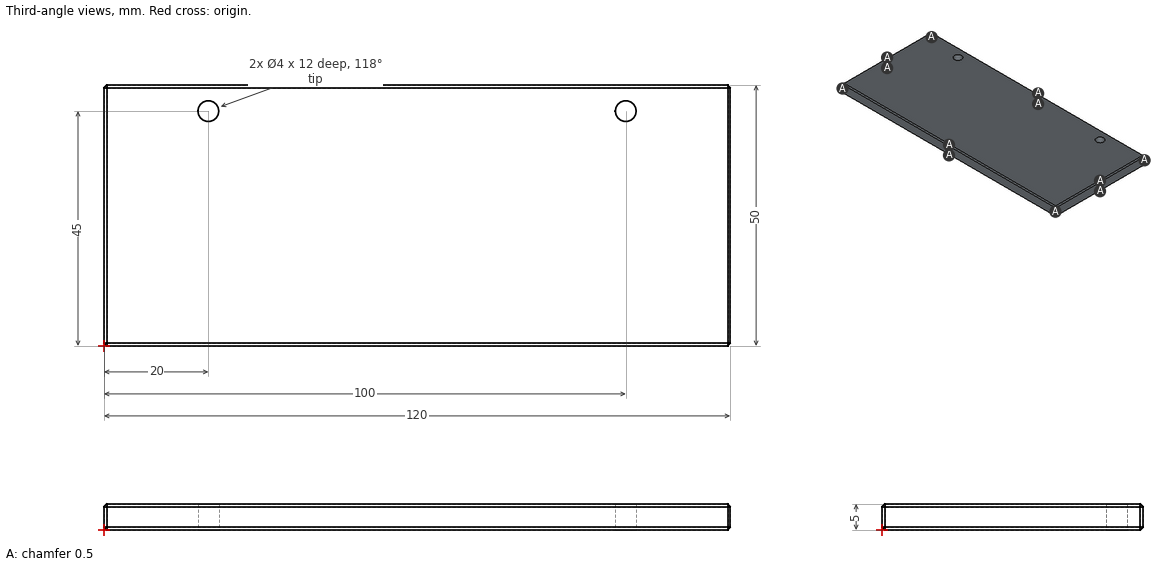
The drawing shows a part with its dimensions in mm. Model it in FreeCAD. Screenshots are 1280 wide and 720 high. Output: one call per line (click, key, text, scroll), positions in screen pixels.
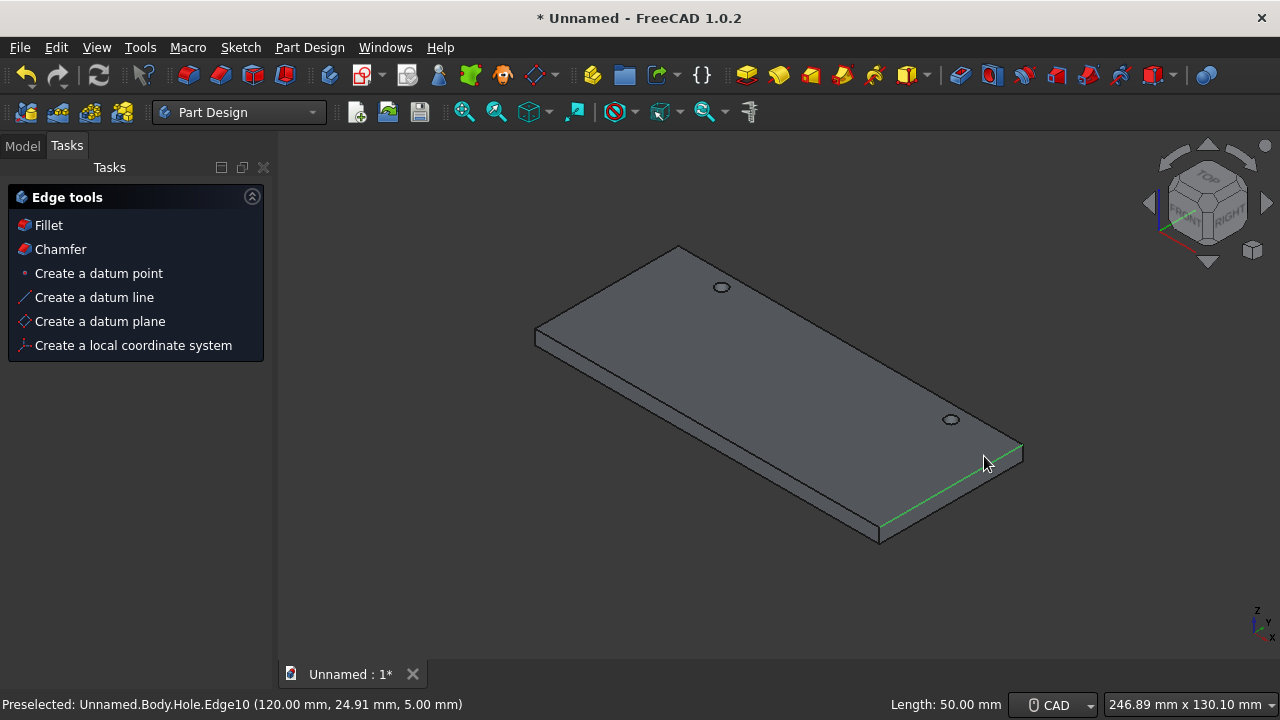
key(2)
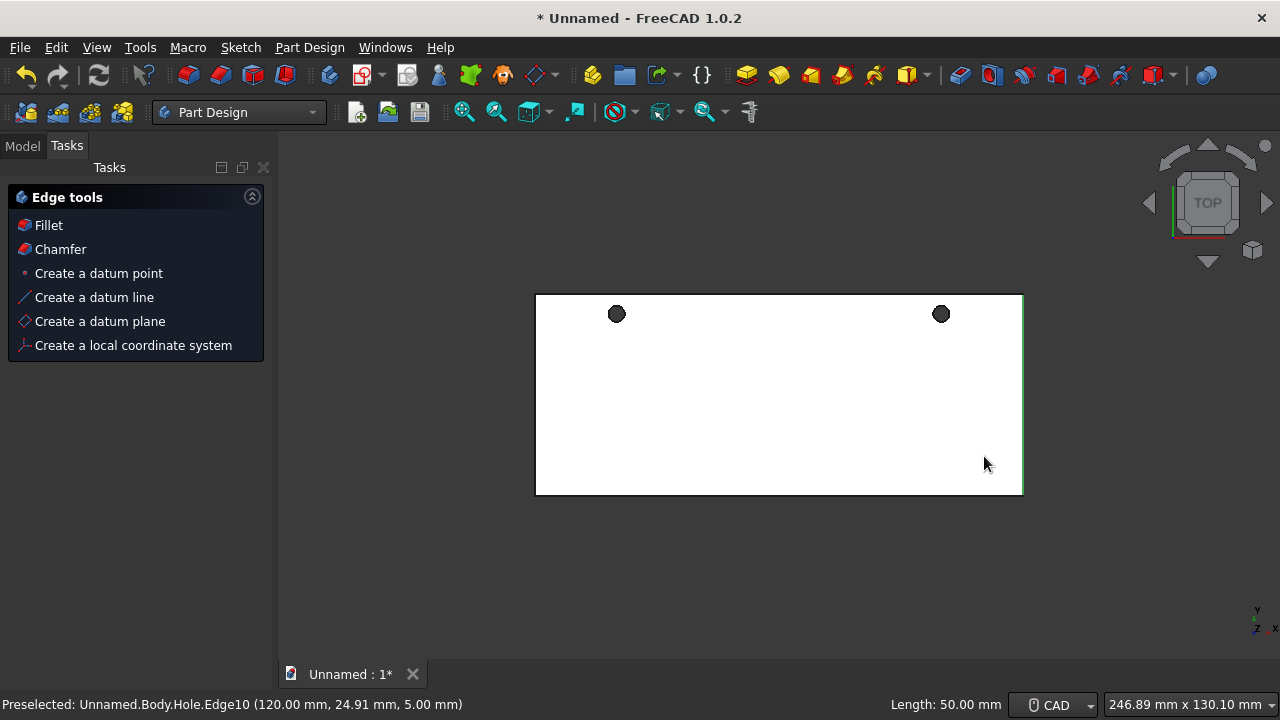
click(535, 394, ctrl)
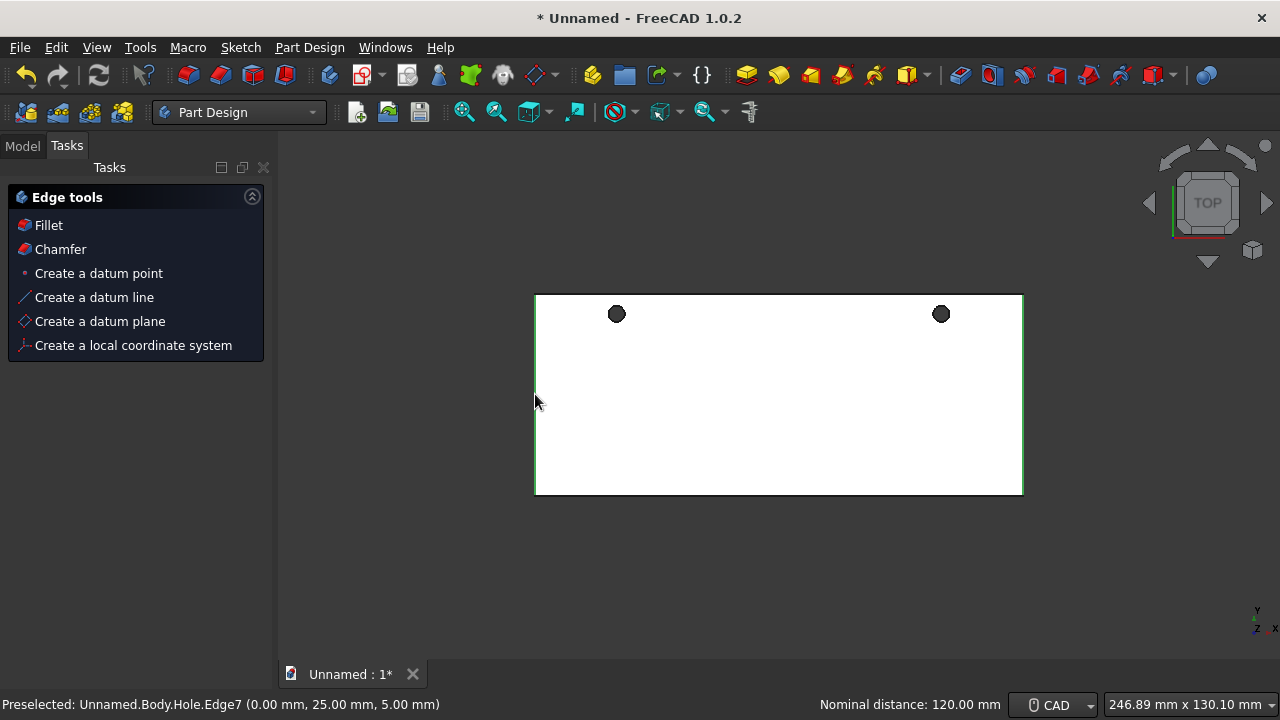
key(1)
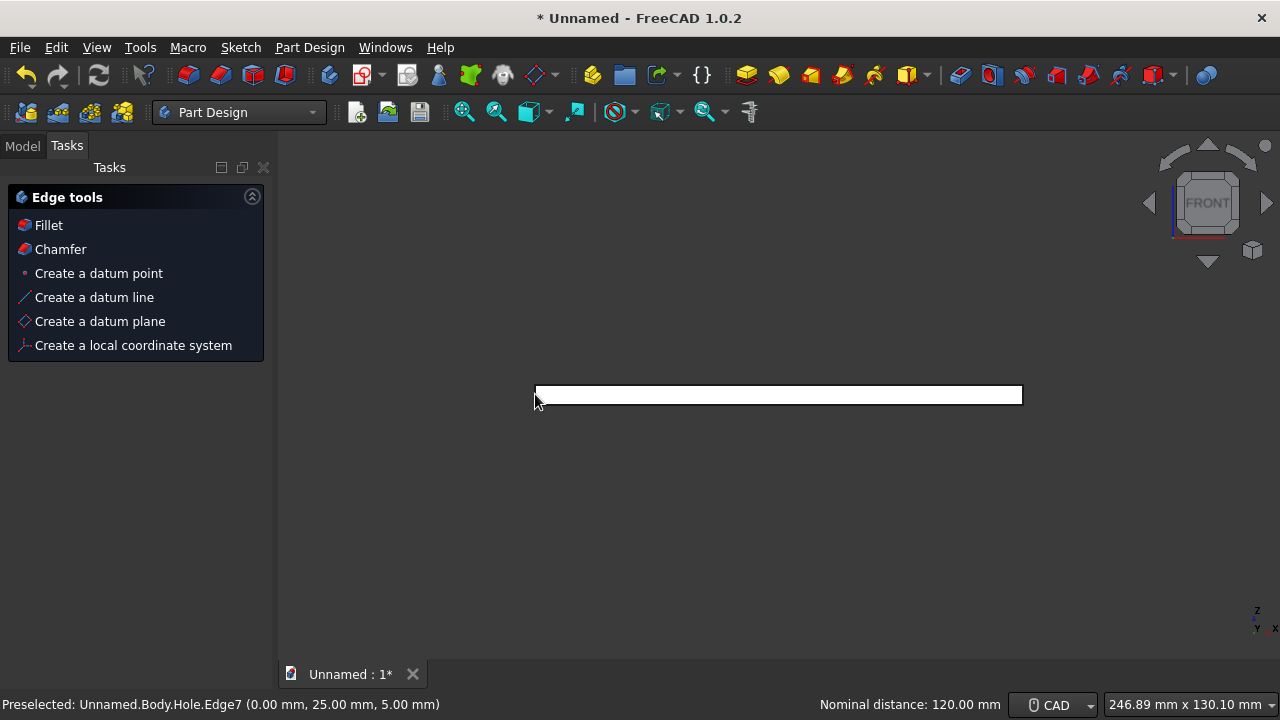
click(988, 394, ctrl)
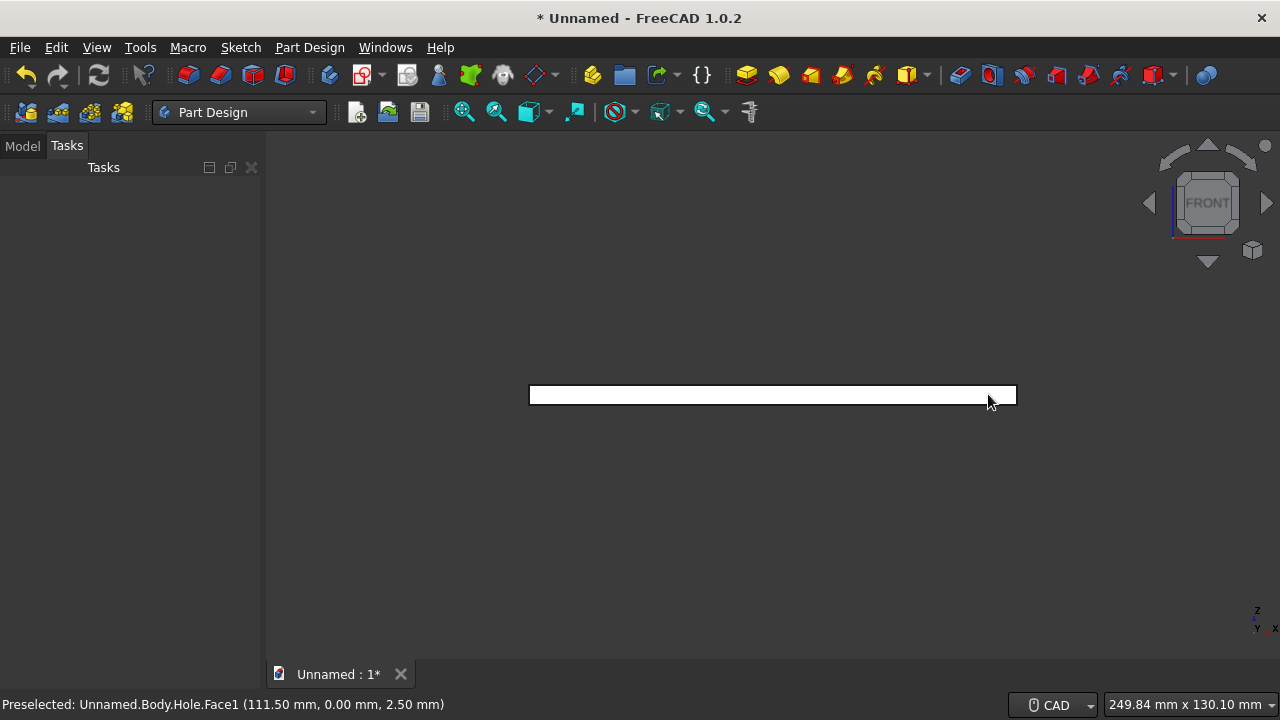
key(3)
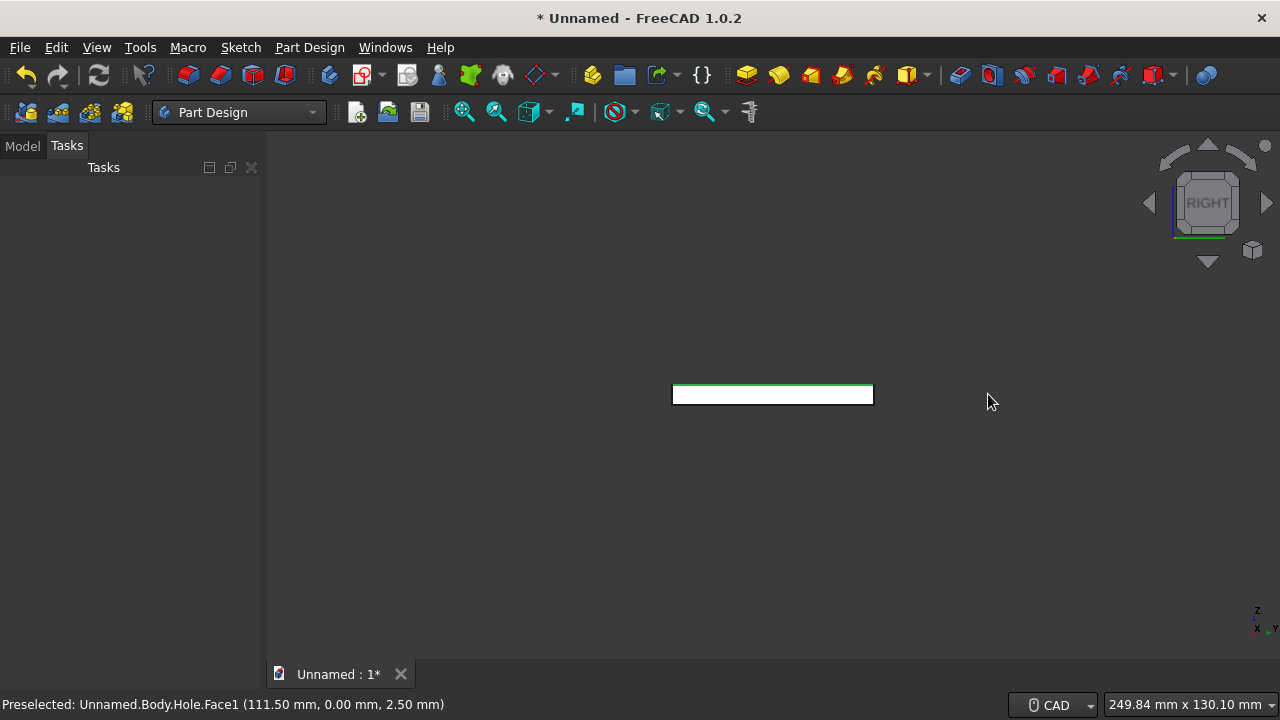
click(466, 112)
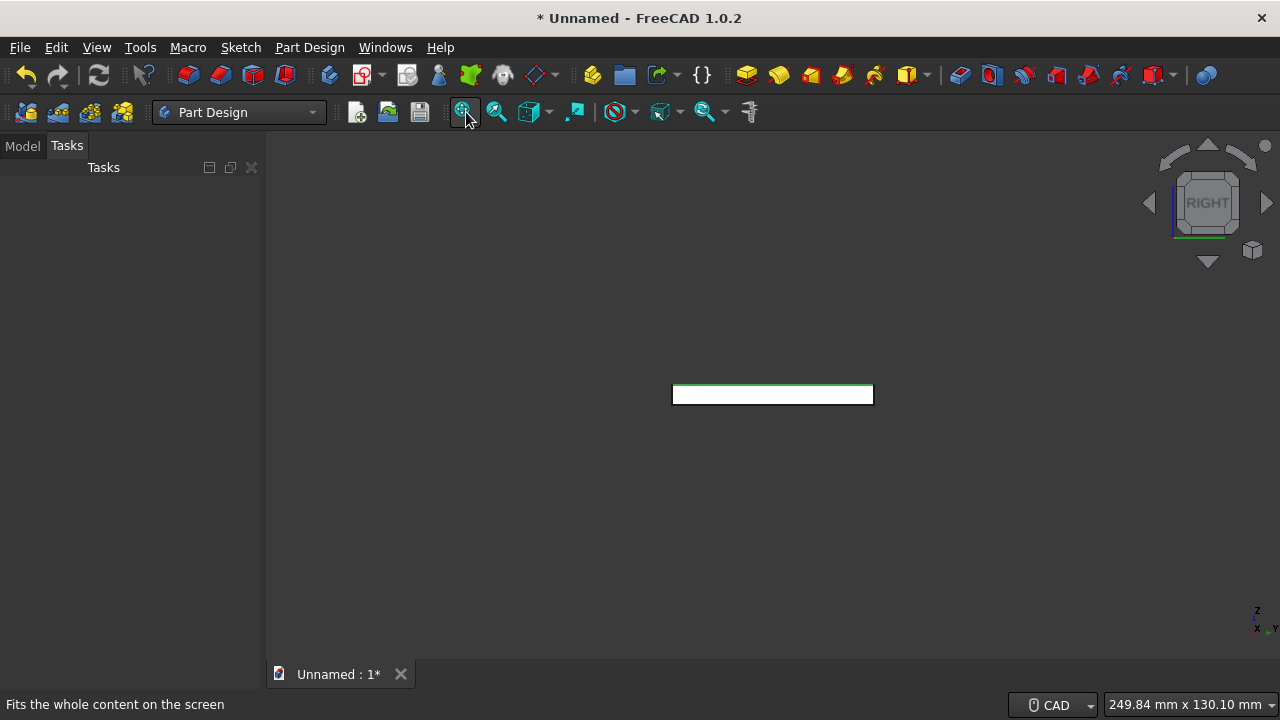
click(773, 404, ctrl)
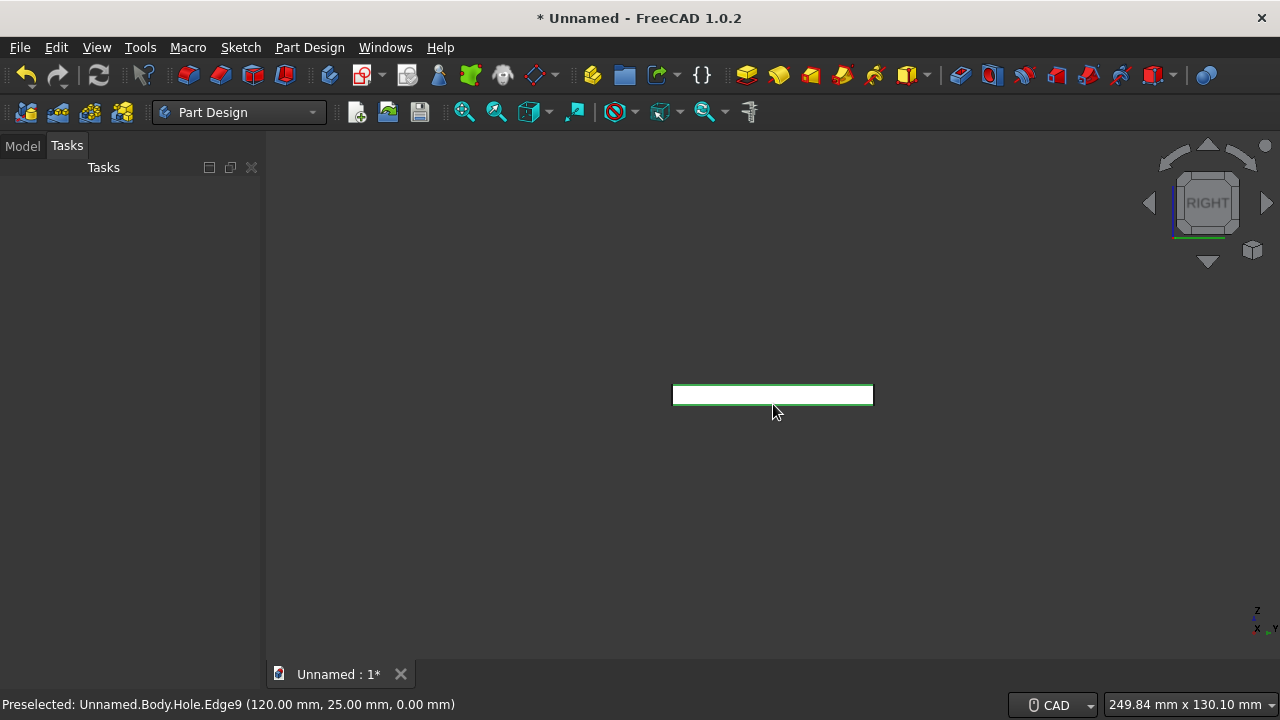
key(5)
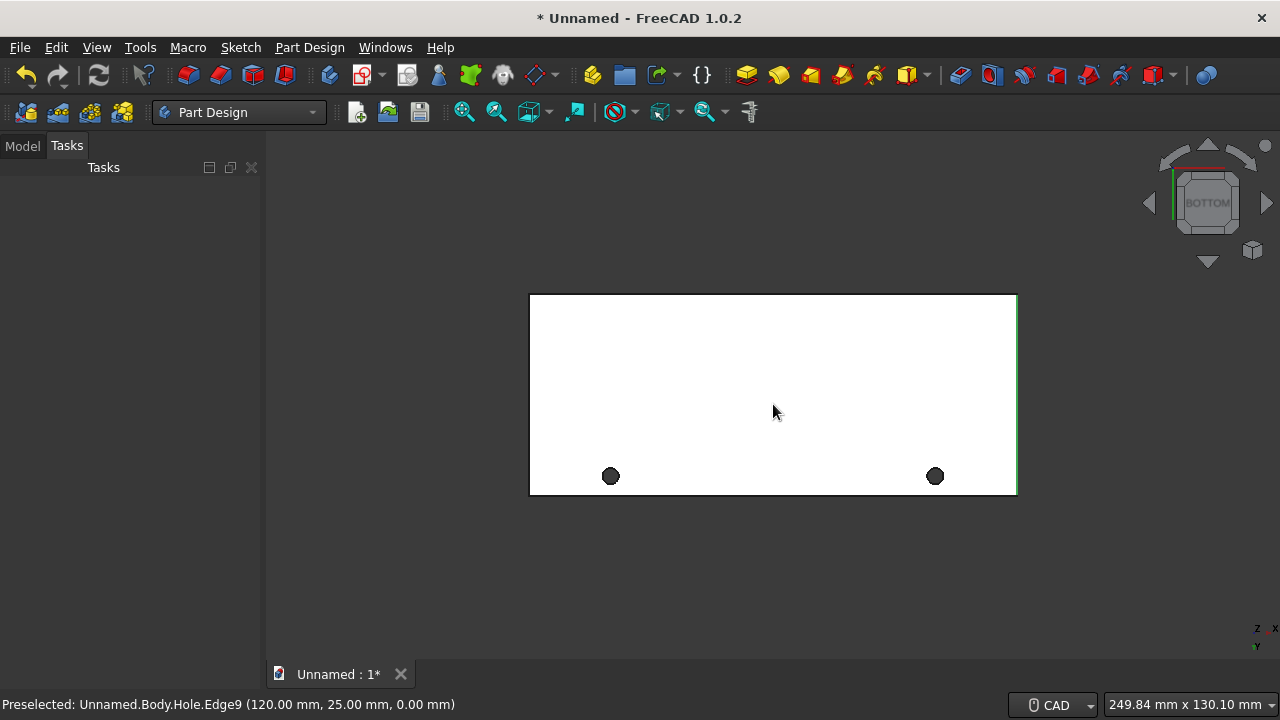
click(529, 394, ctrl)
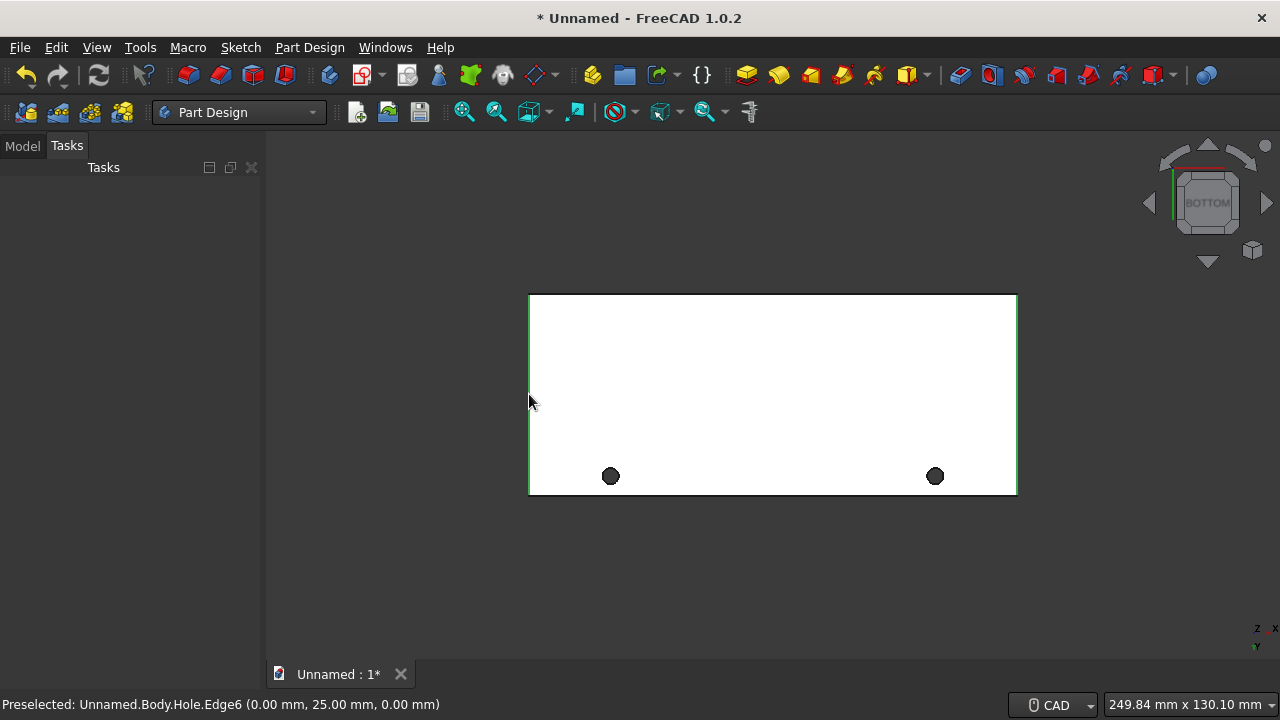
key(4)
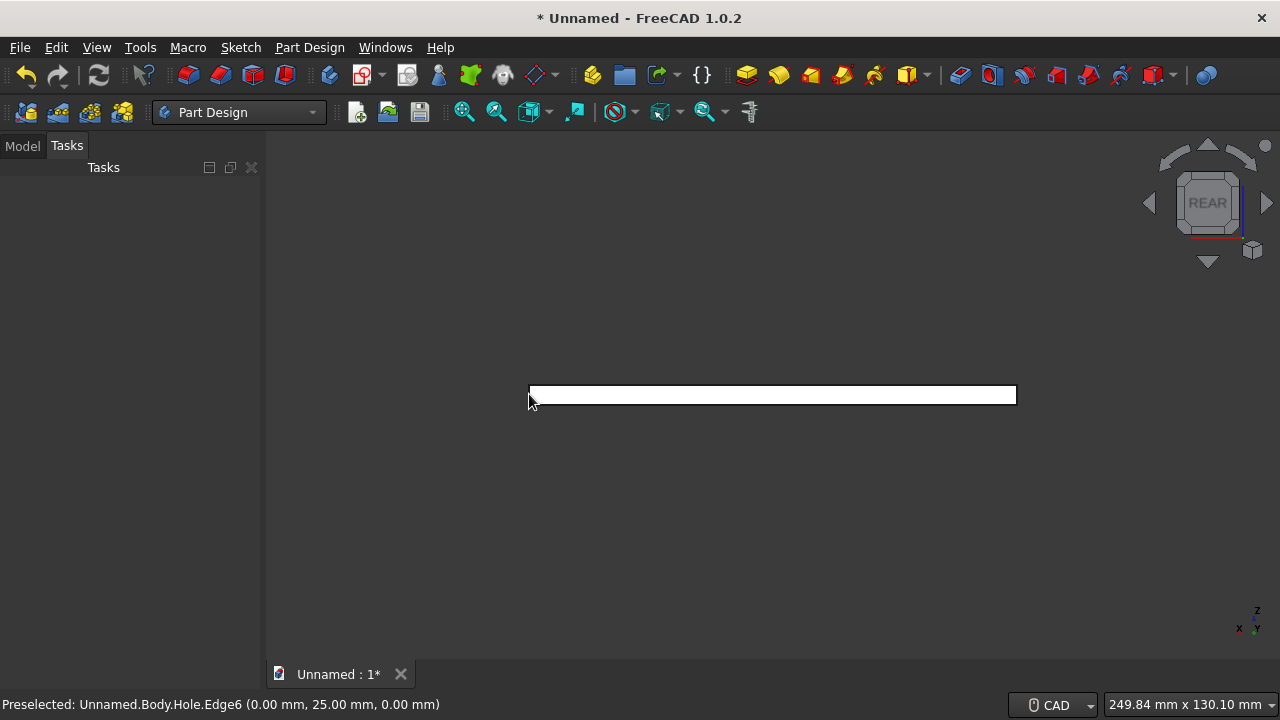
click(564, 394, ctrl)